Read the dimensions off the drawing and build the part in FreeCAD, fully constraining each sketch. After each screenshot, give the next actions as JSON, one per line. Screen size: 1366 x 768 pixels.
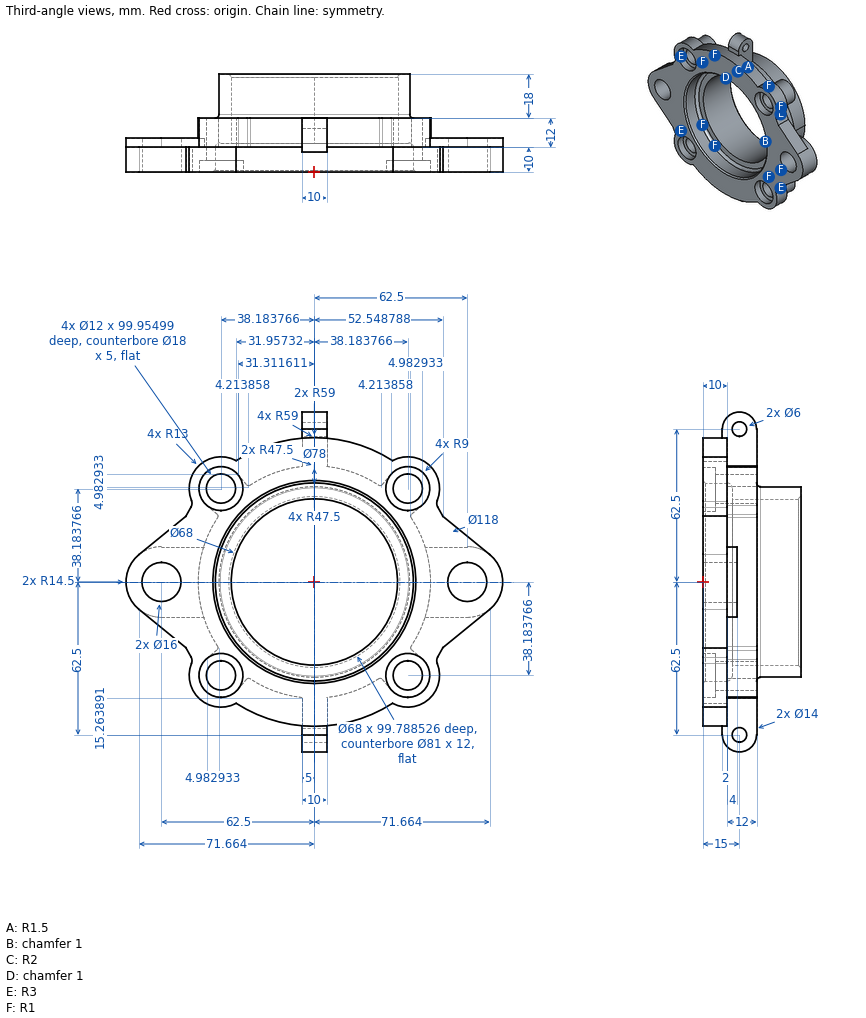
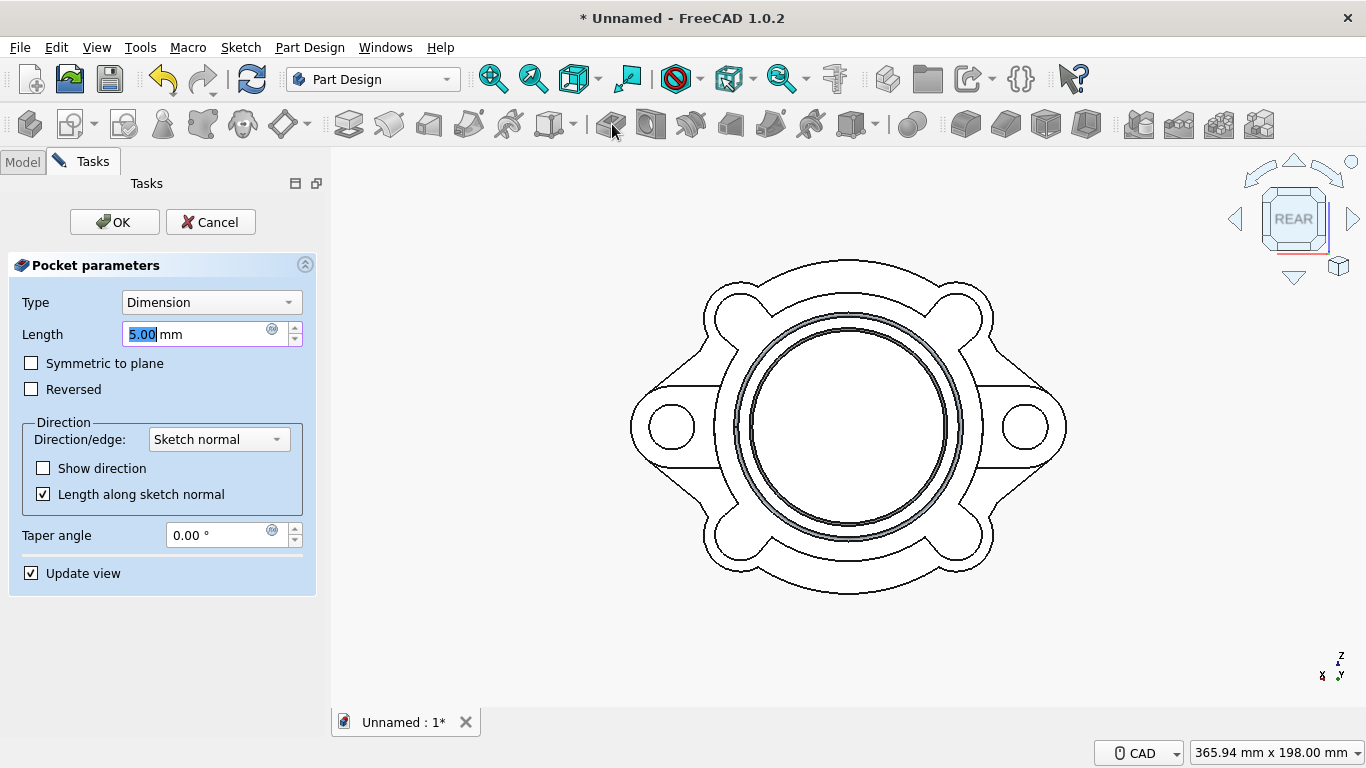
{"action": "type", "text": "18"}
{"action": "key", "text": "Tab"}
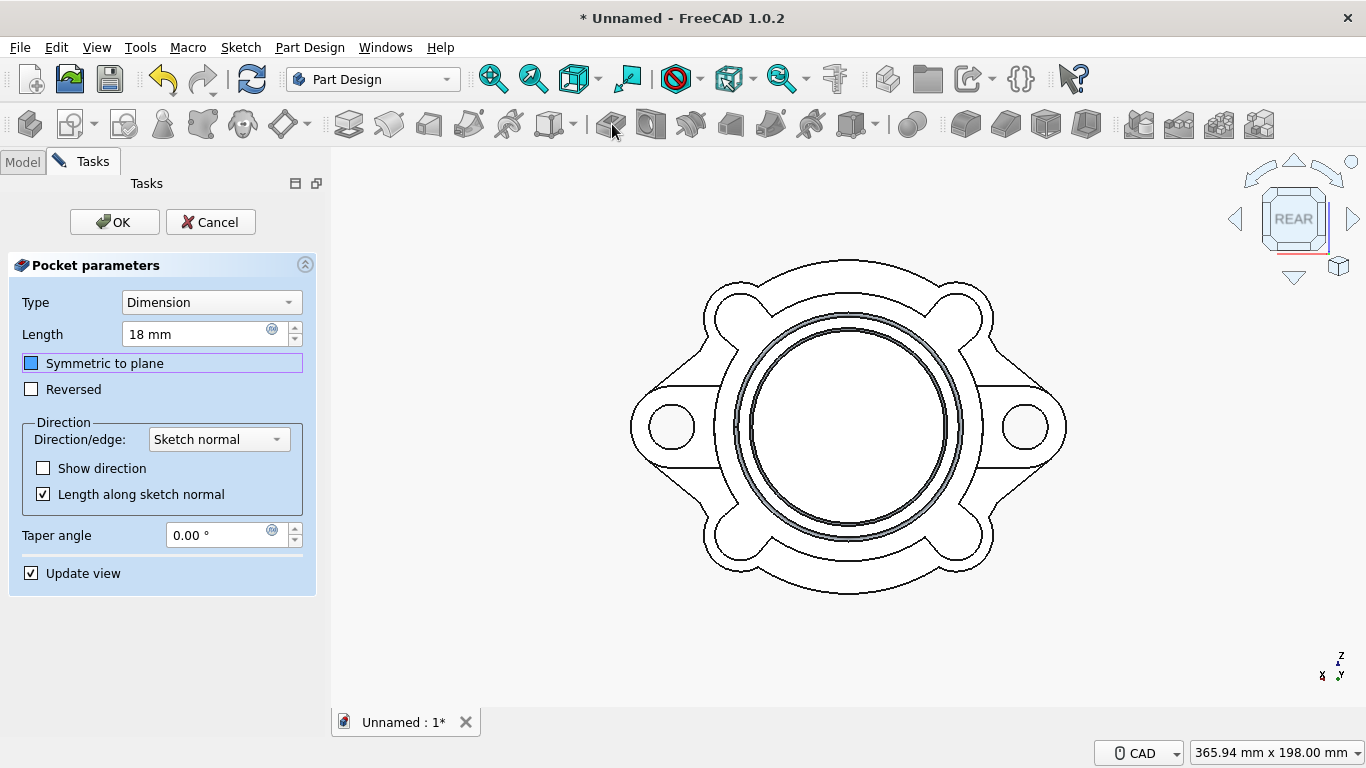
{"action": "left_click", "coordinate": [115, 222]}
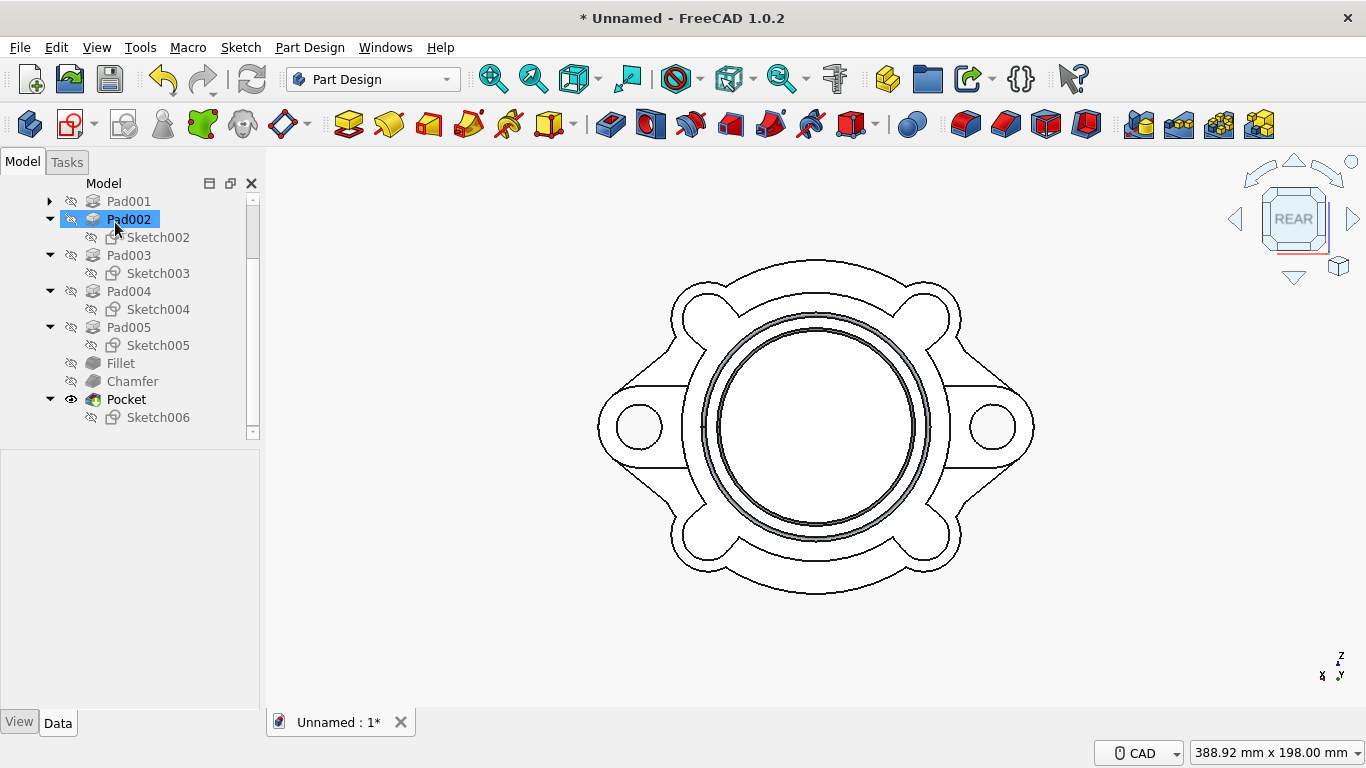
{"action": "left_click", "coordinate": [70, 124]}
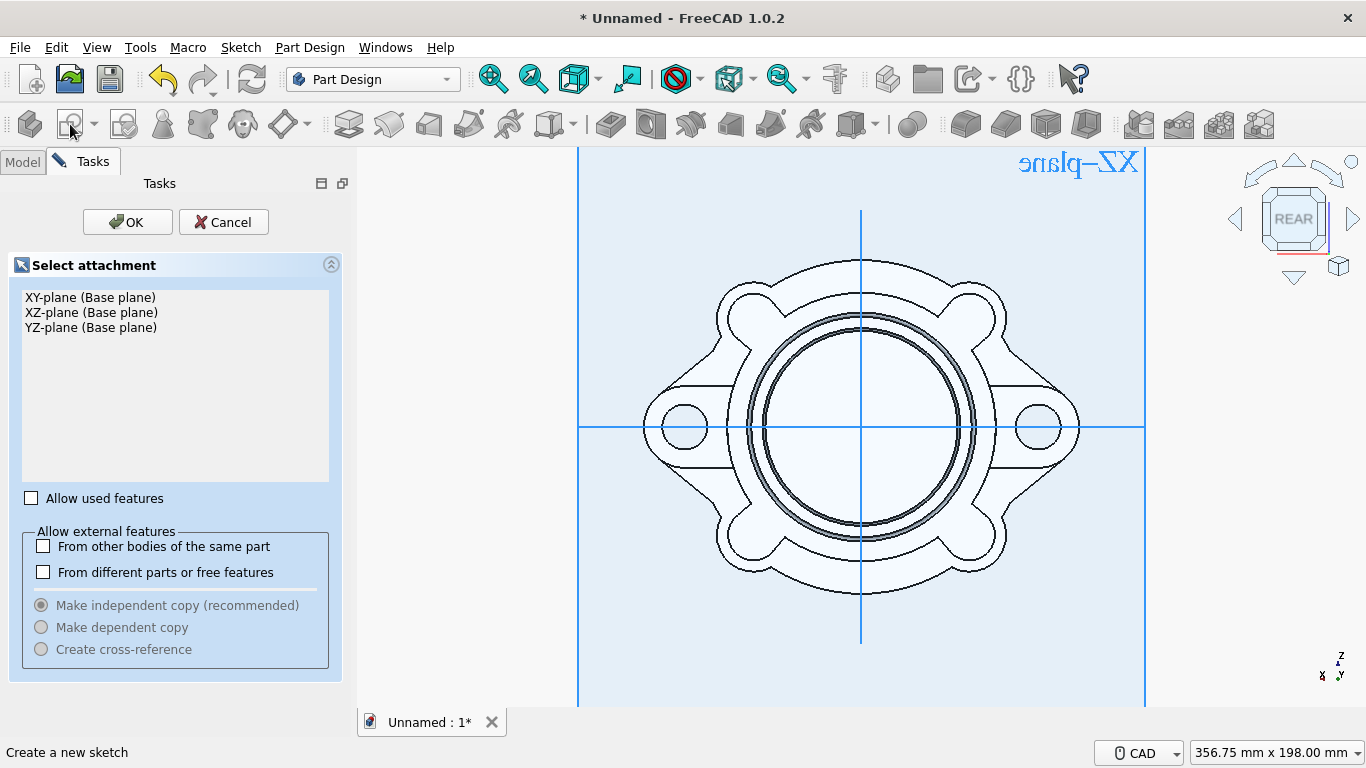
{"action": "left_click", "coordinate": [82, 312]}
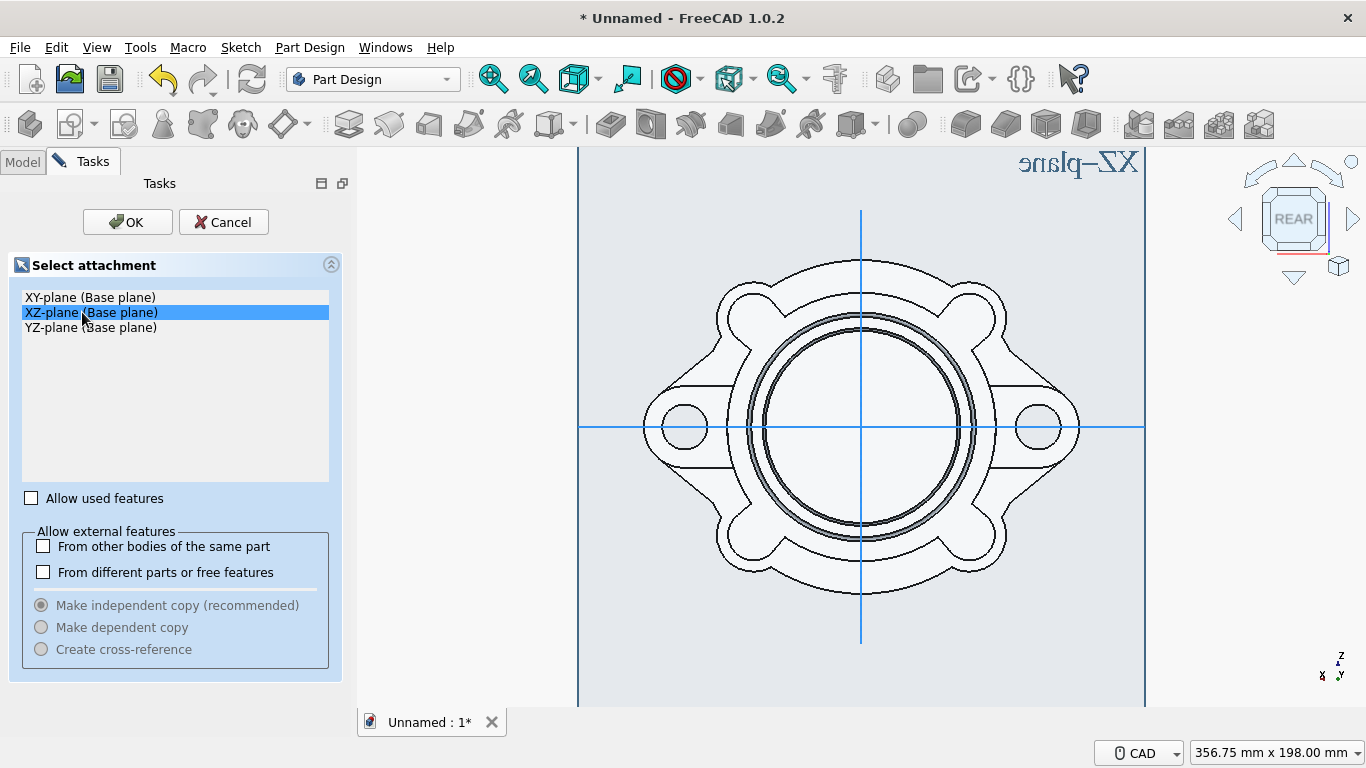
{"action": "left_click", "coordinate": [128, 222]}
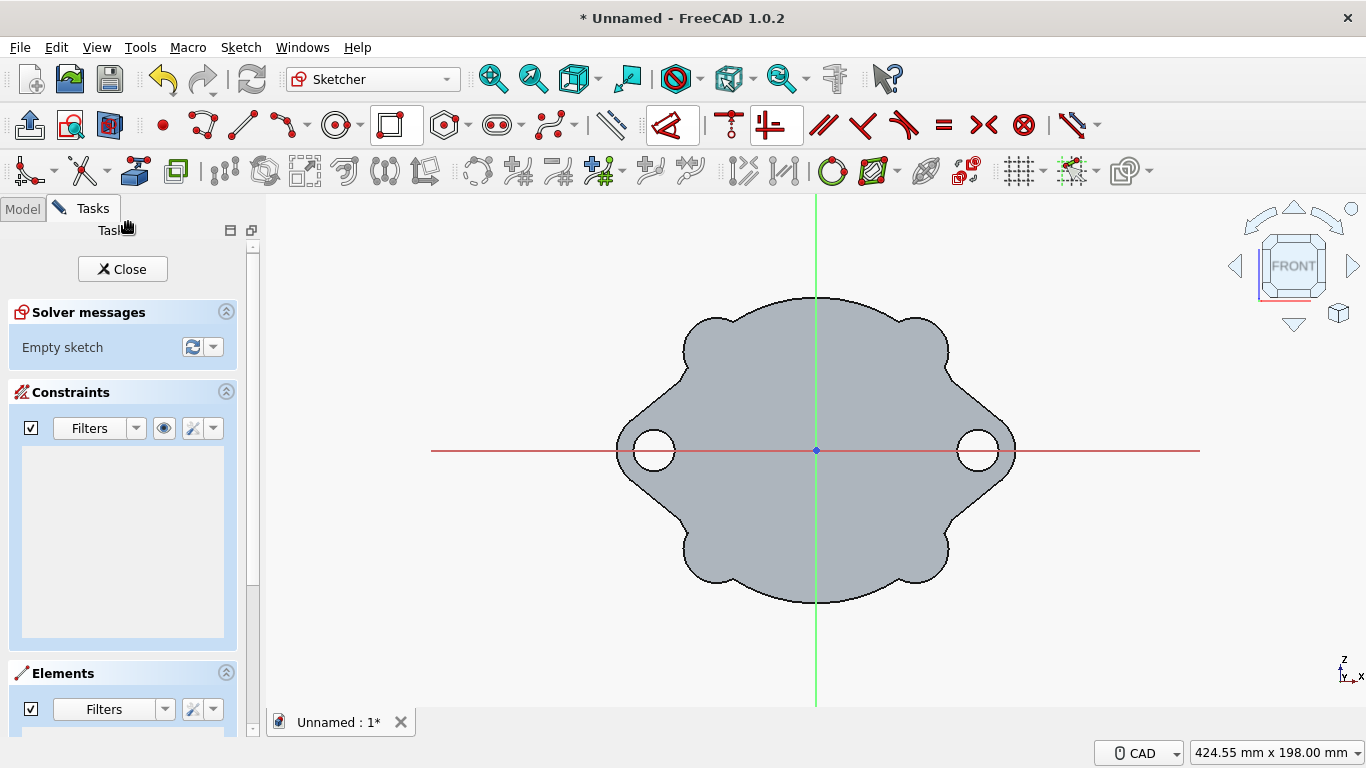
{"action": "scroll", "coordinate": [955, 451], "scroll_direction": "up", "scroll_amount": 2}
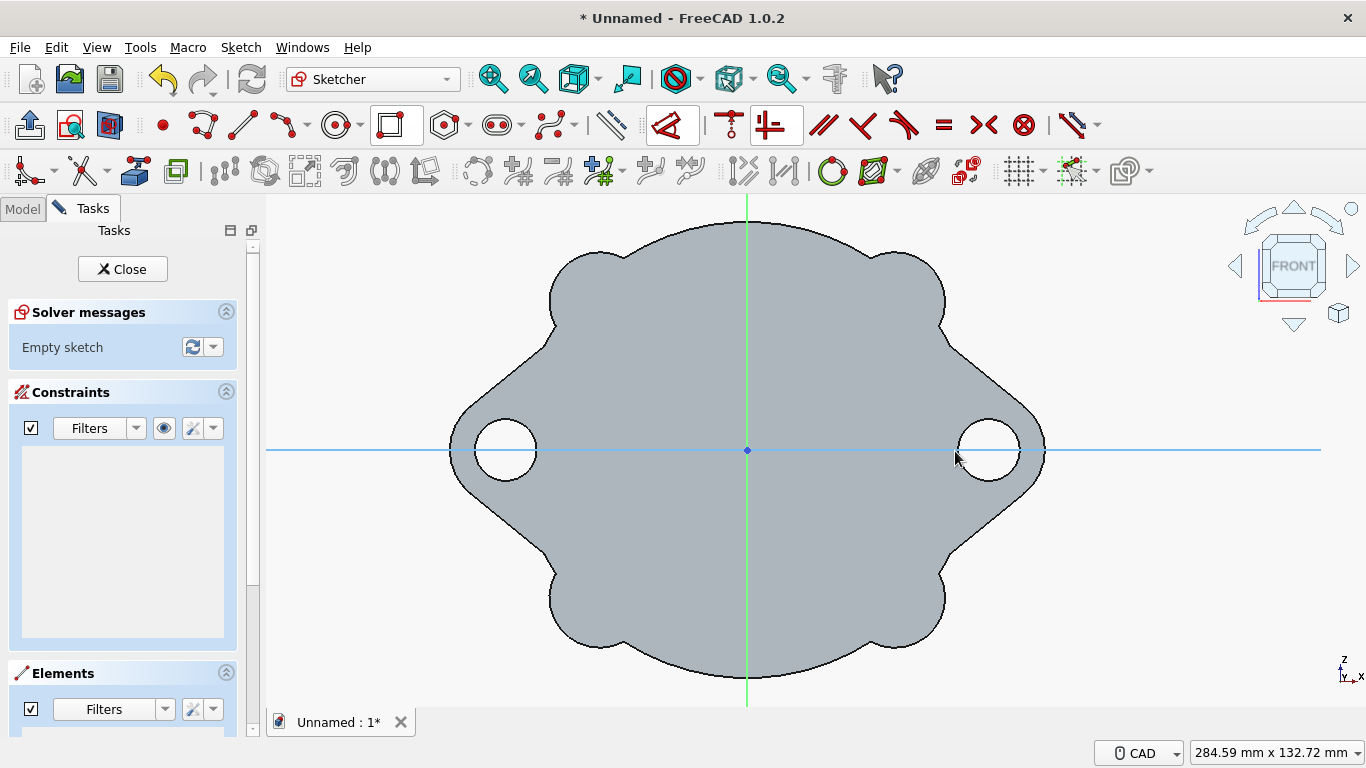
{"action": "left_click", "coordinate": [336, 126]}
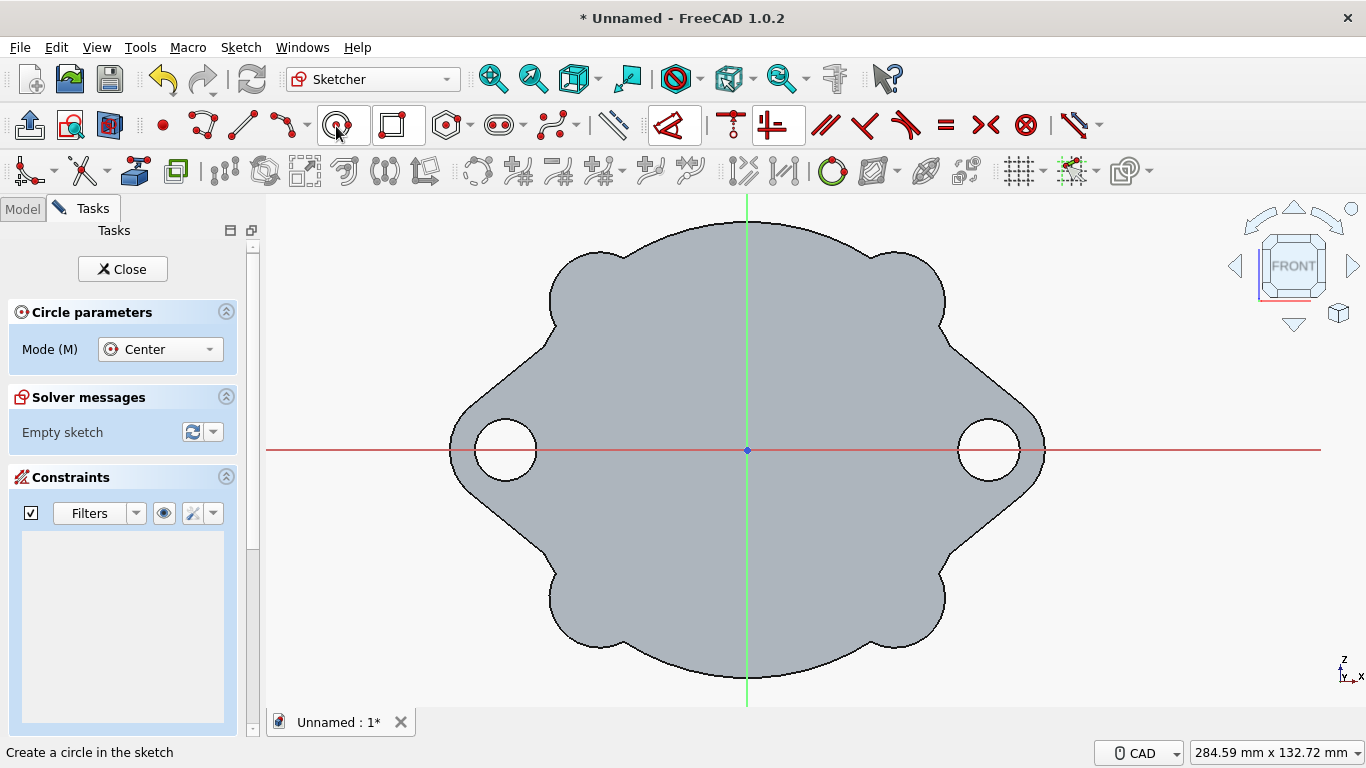
{"action": "left_click", "coordinate": [600, 302]}
{"action": "left_click", "coordinate": [616, 286]}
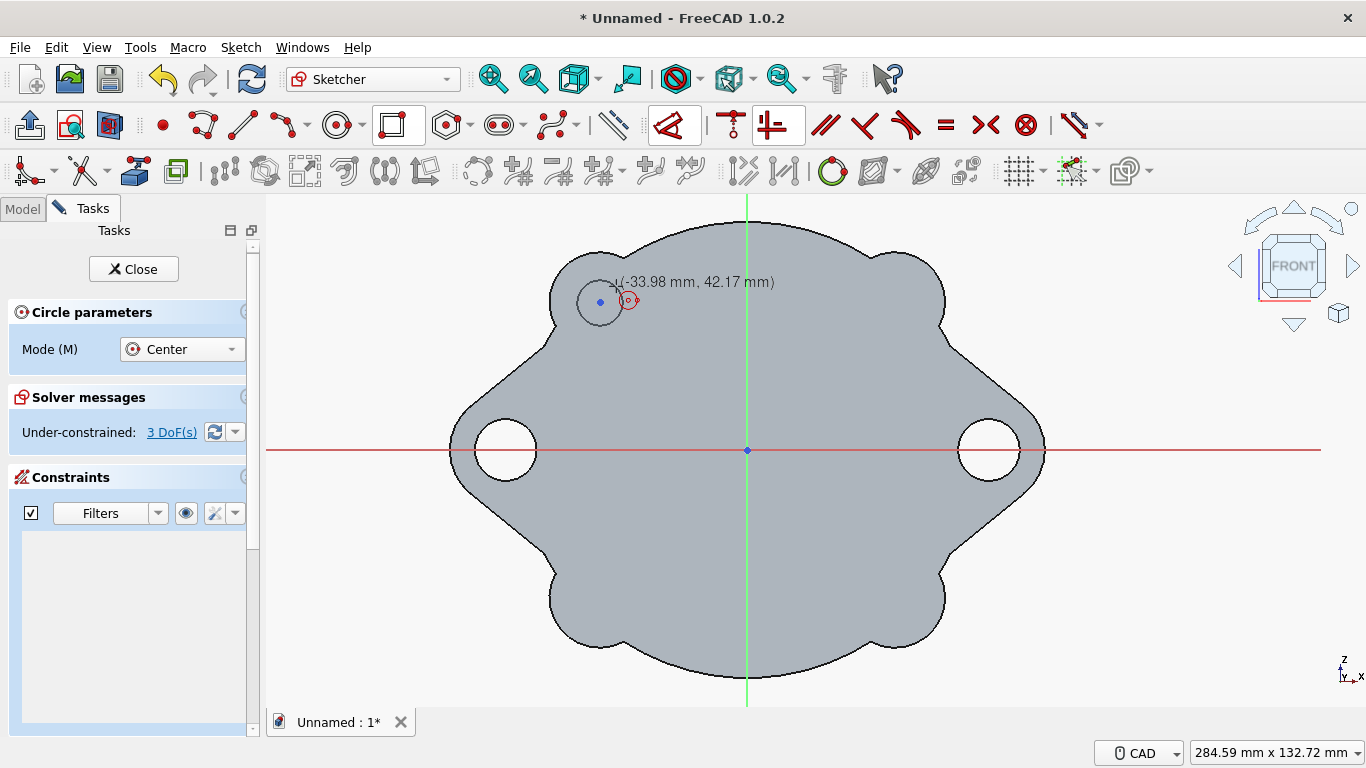
{"action": "left_click", "coordinate": [895, 302]}
{"action": "left_click", "coordinate": [911, 286]}